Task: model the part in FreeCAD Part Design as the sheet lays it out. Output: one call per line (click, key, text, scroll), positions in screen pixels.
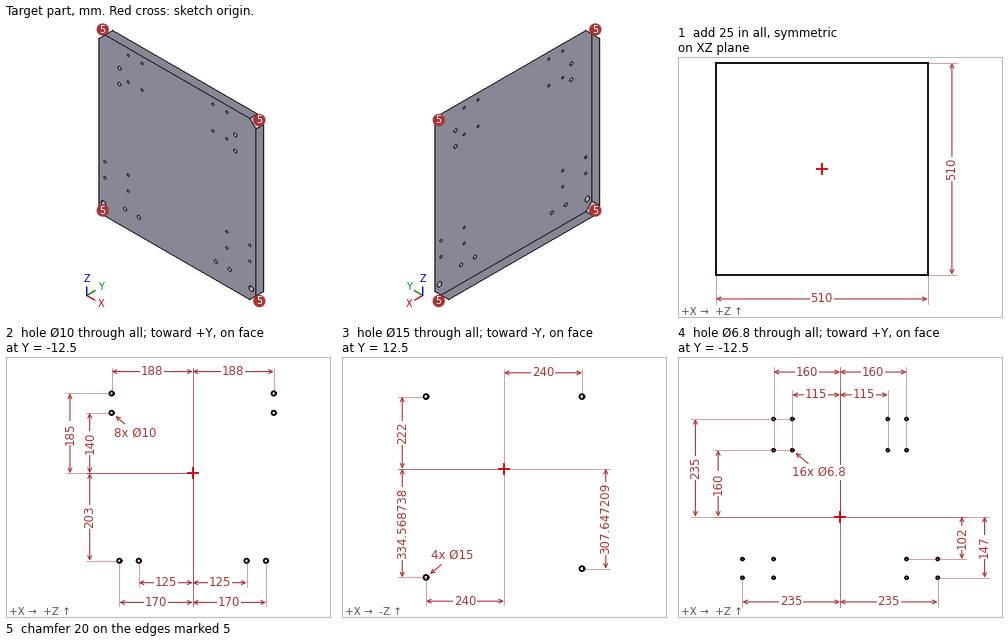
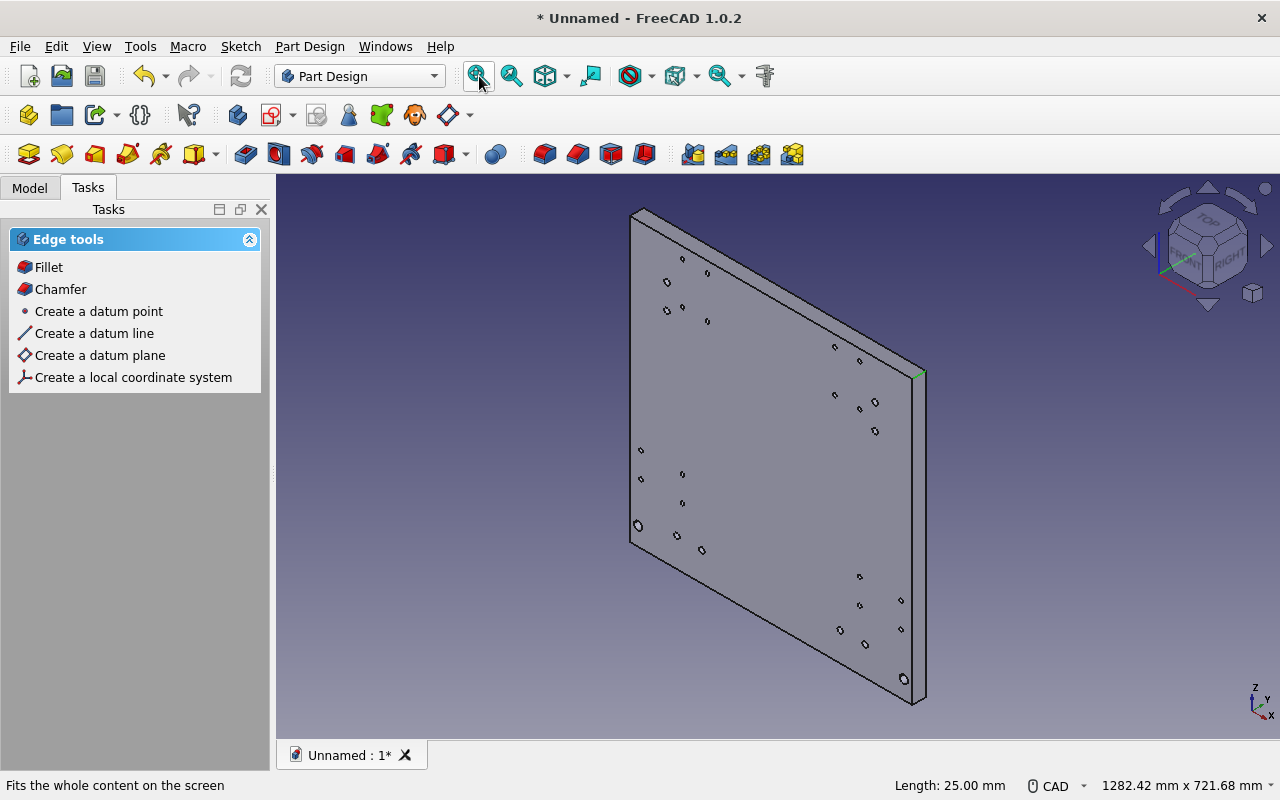
key(2)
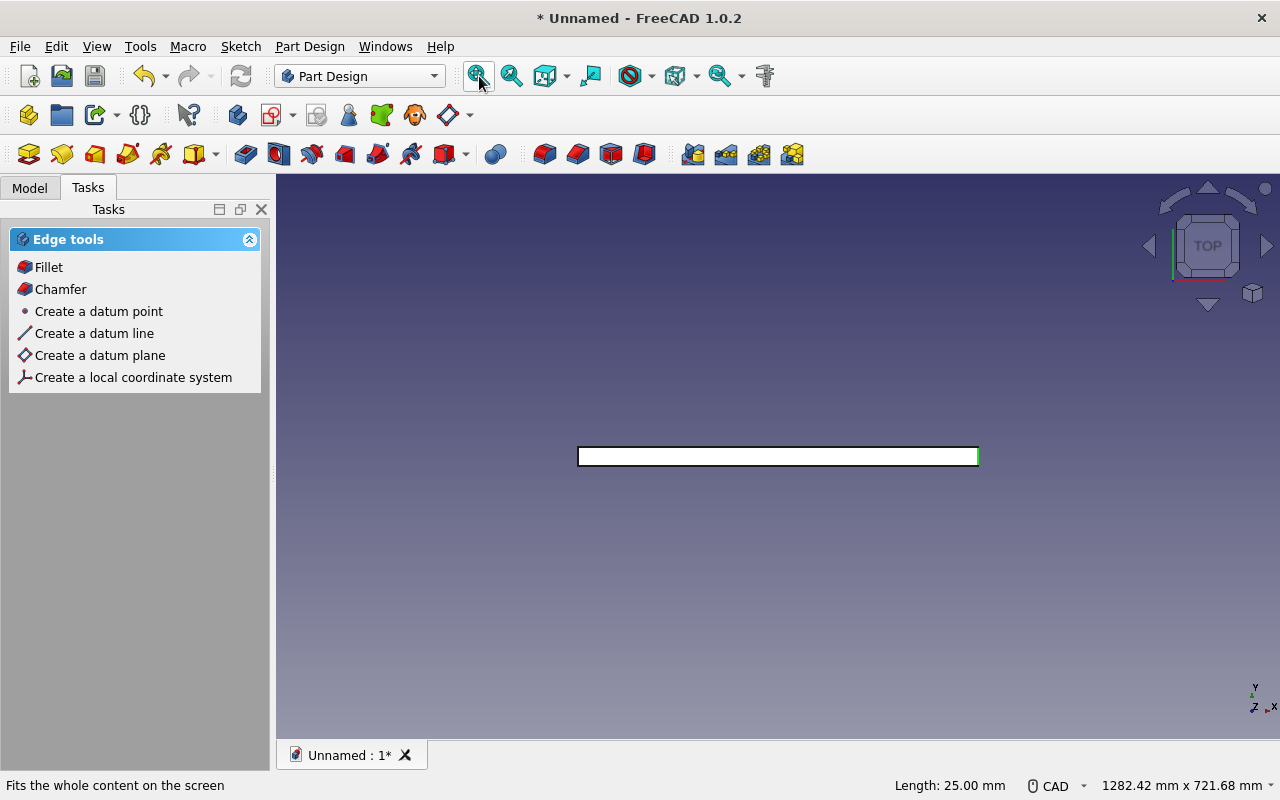
click(479, 76)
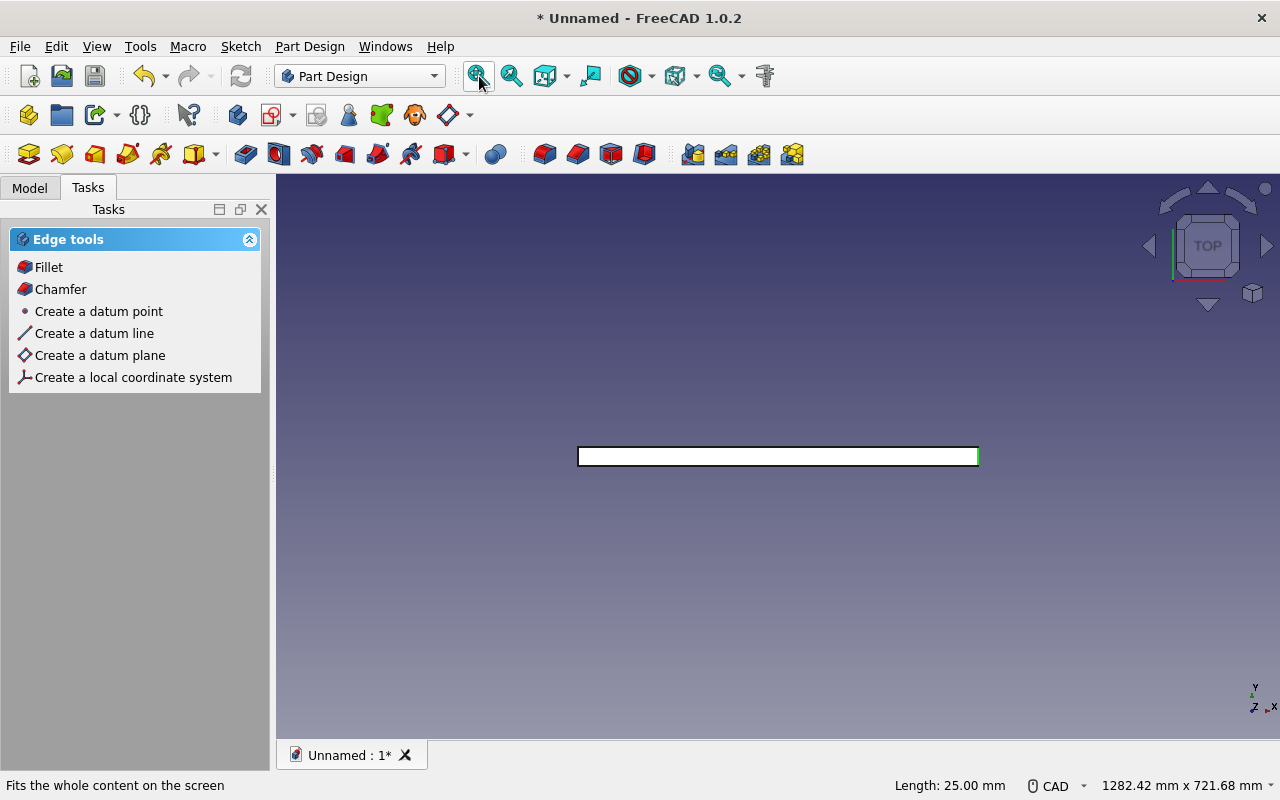
click(578, 455, ctrl)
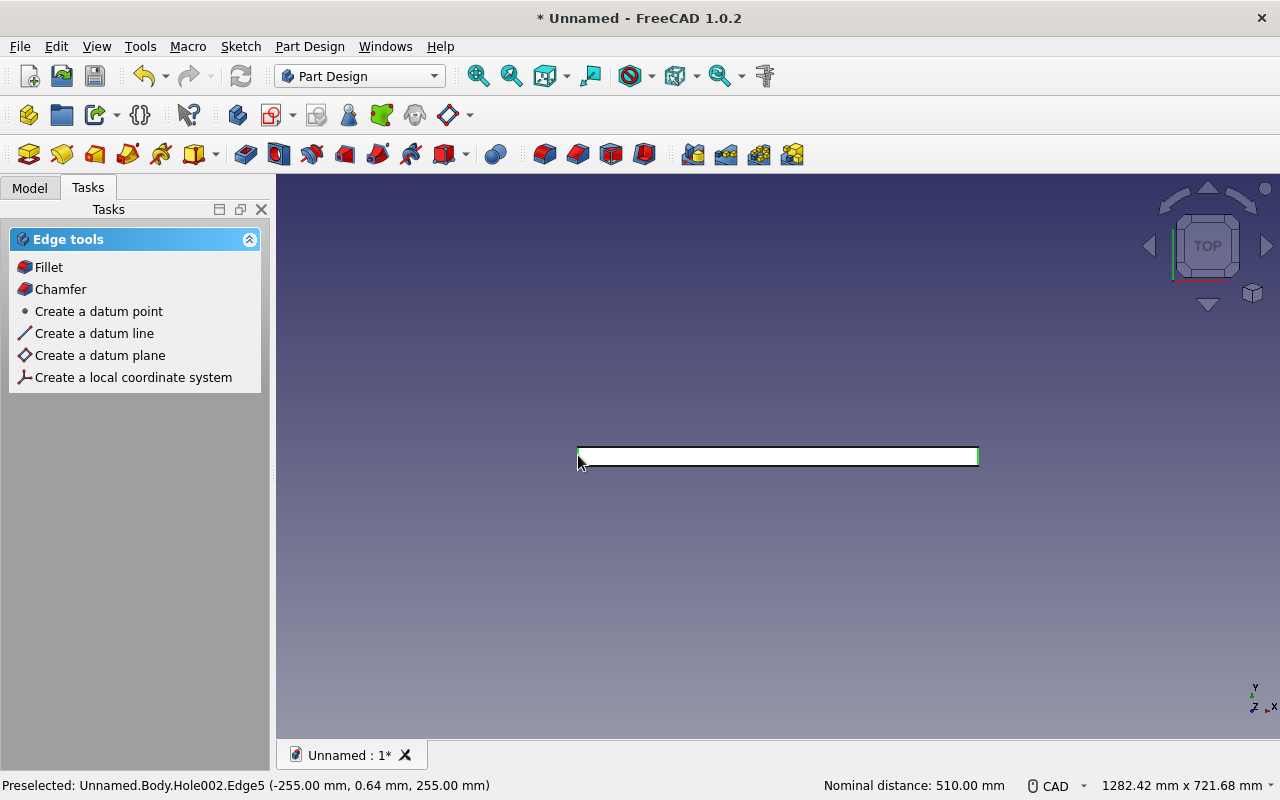
scroll(578, 455, up, 4)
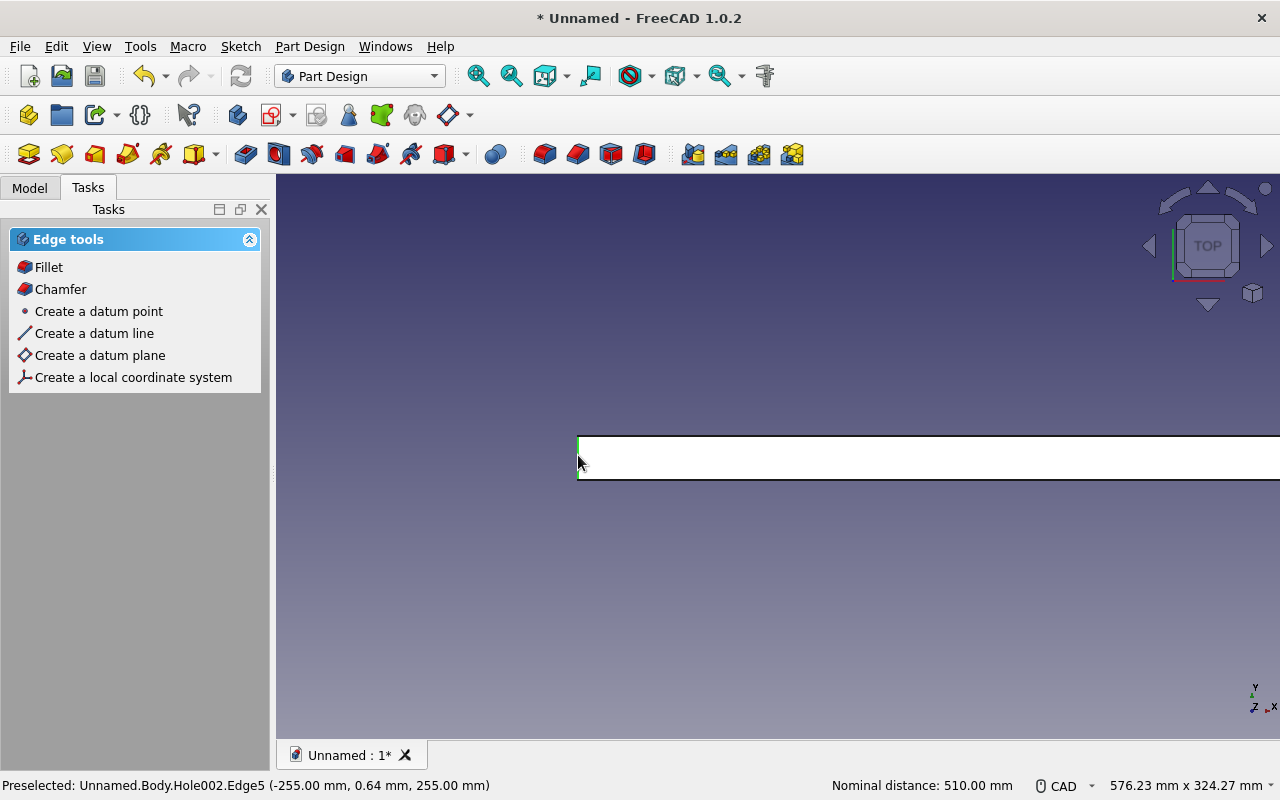
key(v)
key(f)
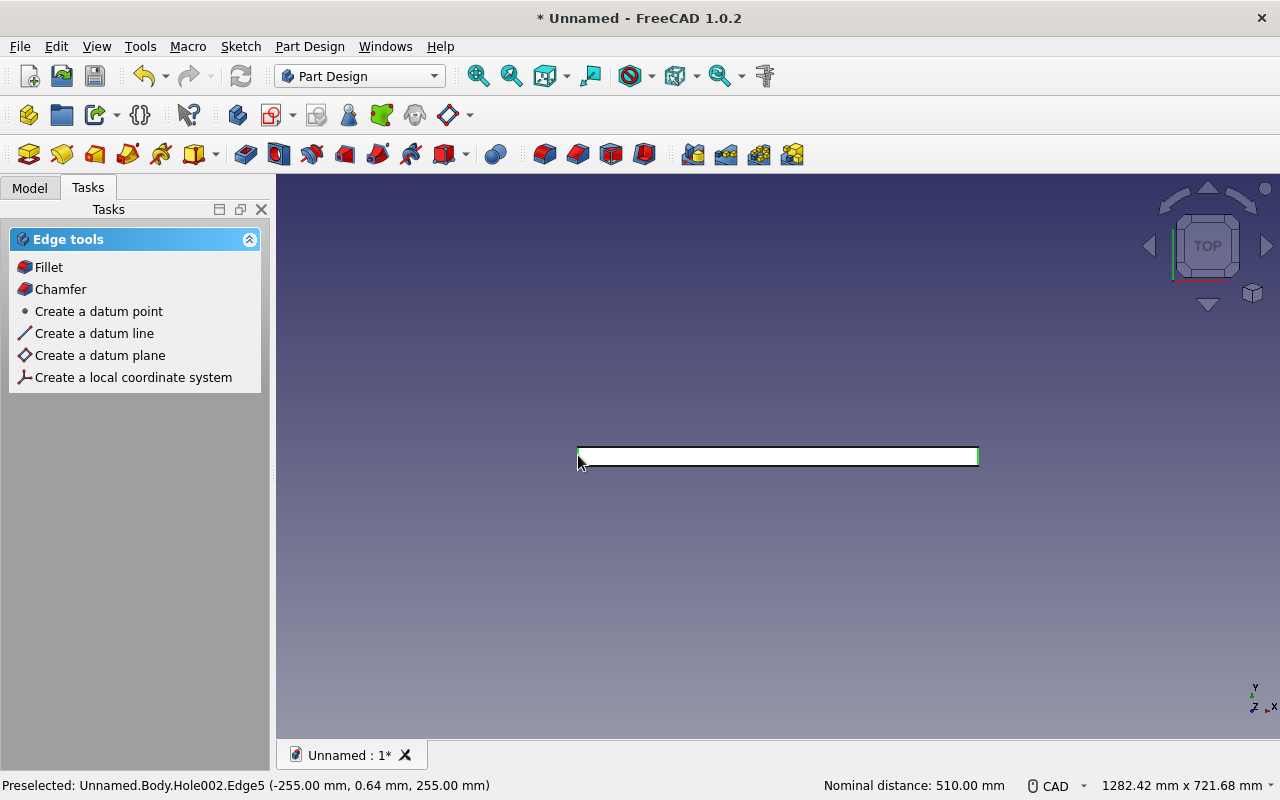
key(0)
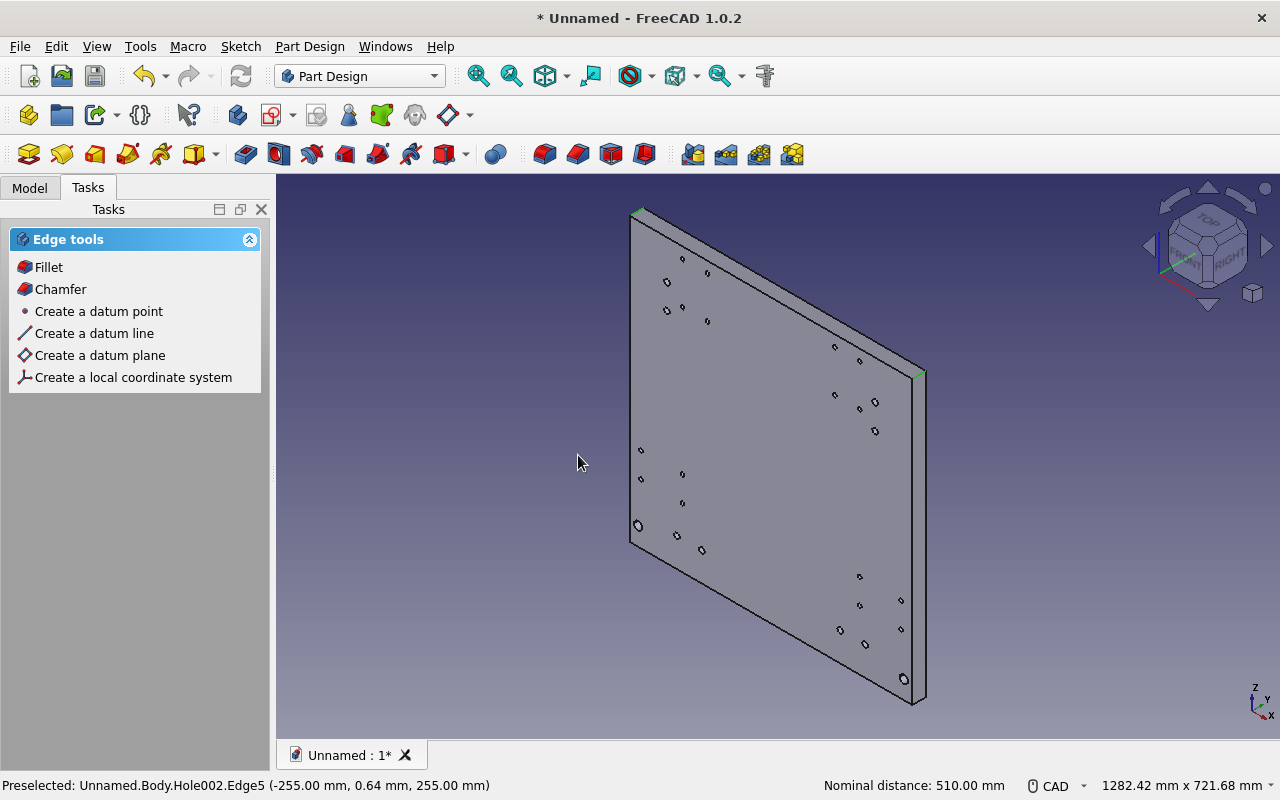
scroll(637, 537, up, 4)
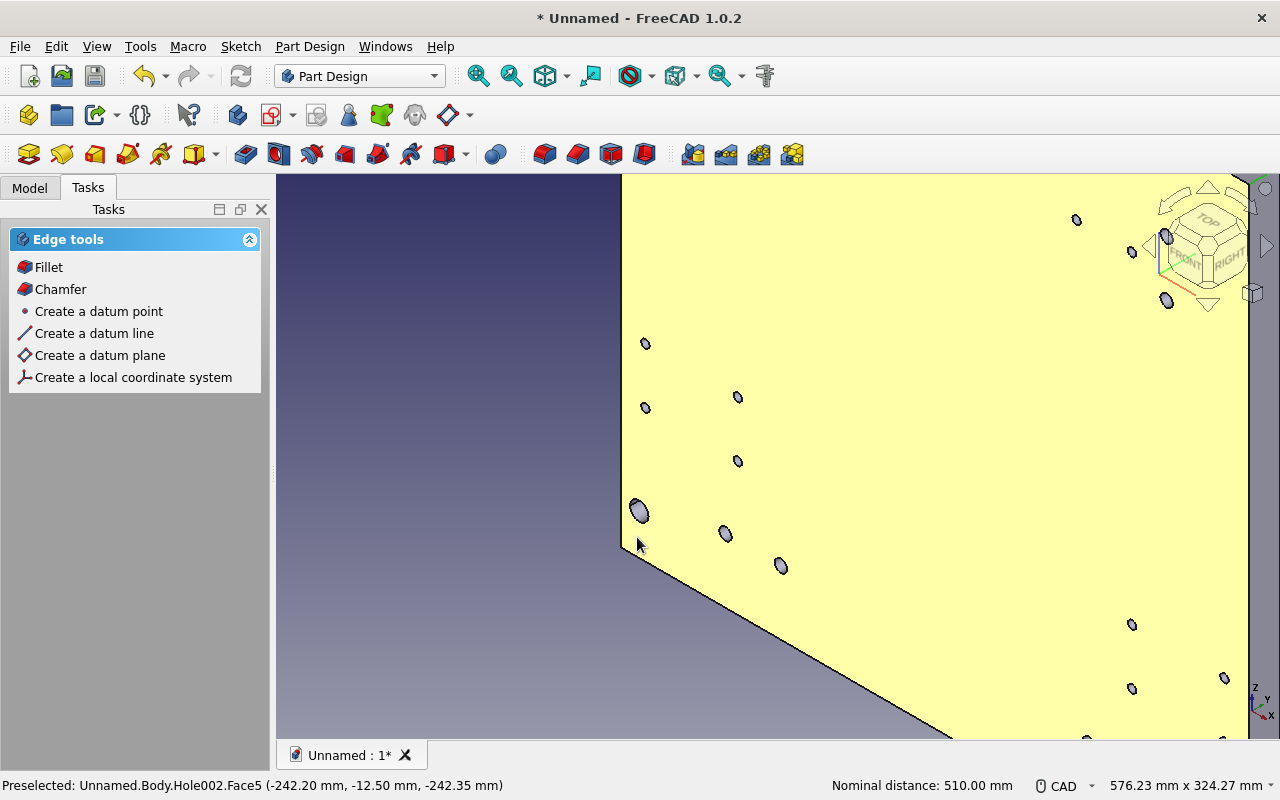
click(479, 76)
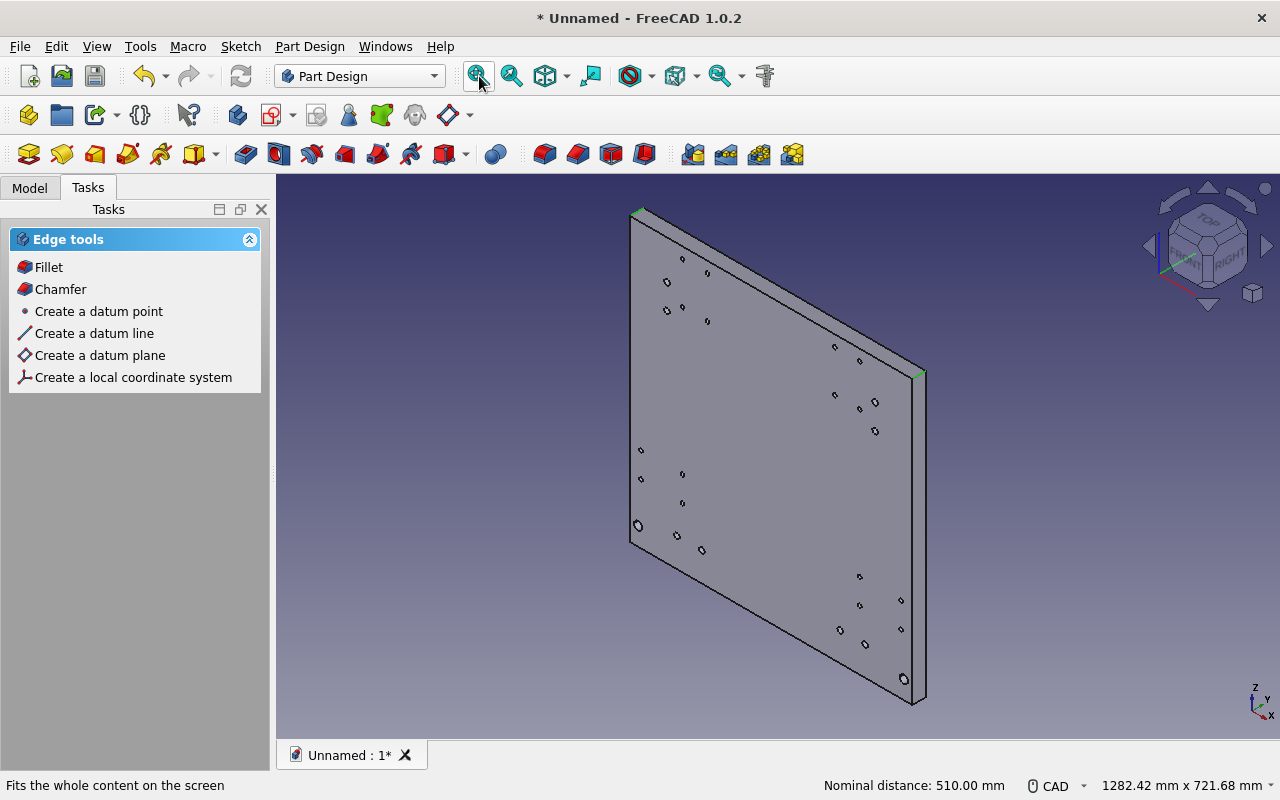
key(1)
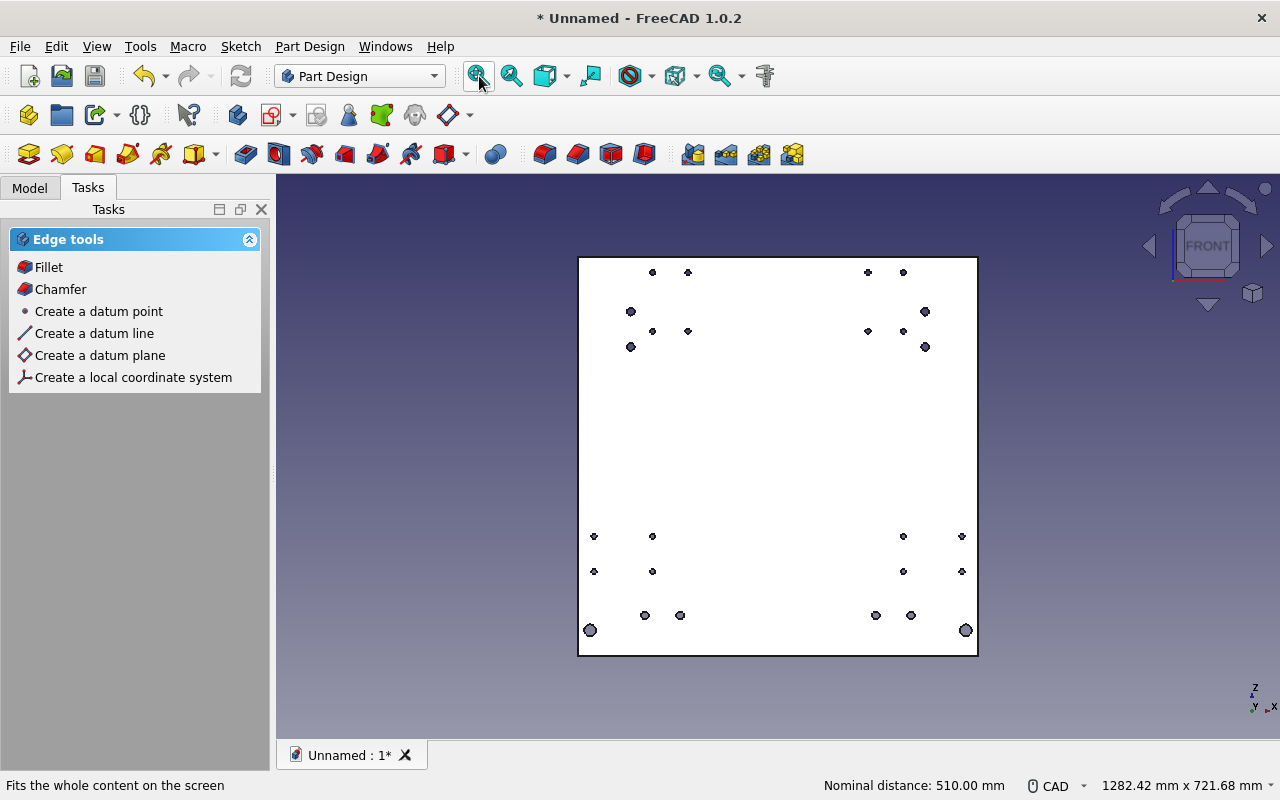
scroll(578, 655, up, 4)